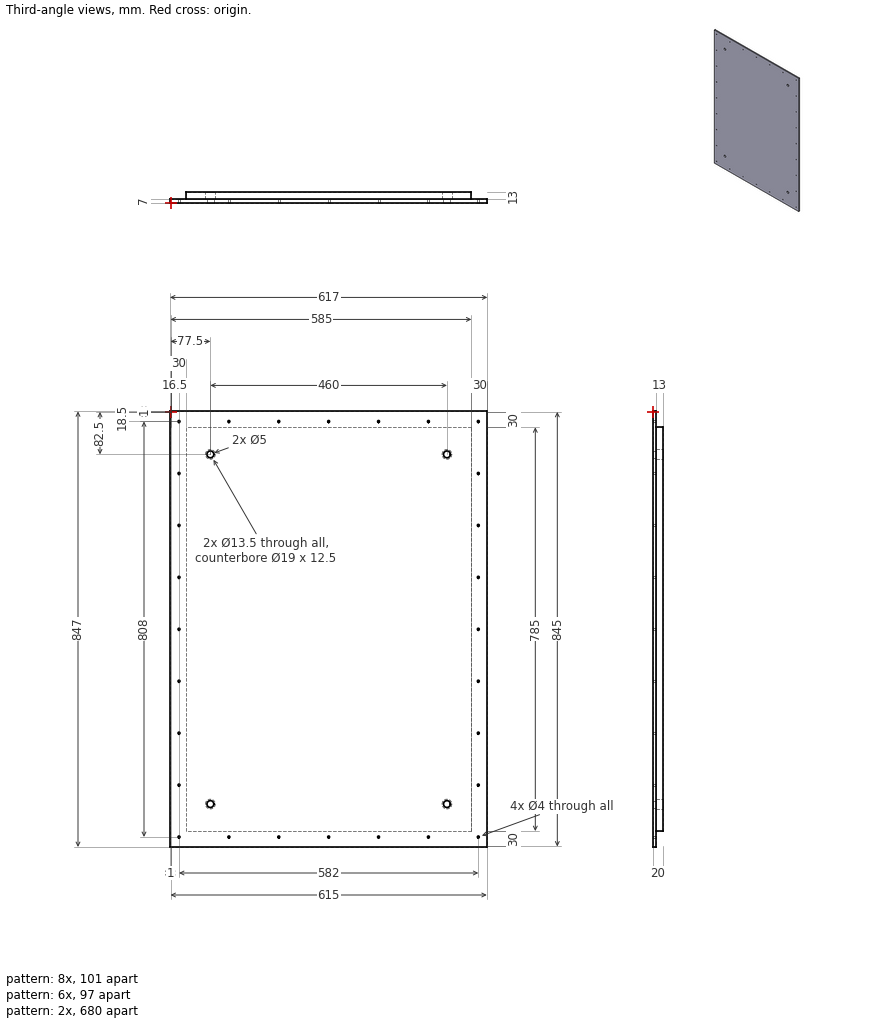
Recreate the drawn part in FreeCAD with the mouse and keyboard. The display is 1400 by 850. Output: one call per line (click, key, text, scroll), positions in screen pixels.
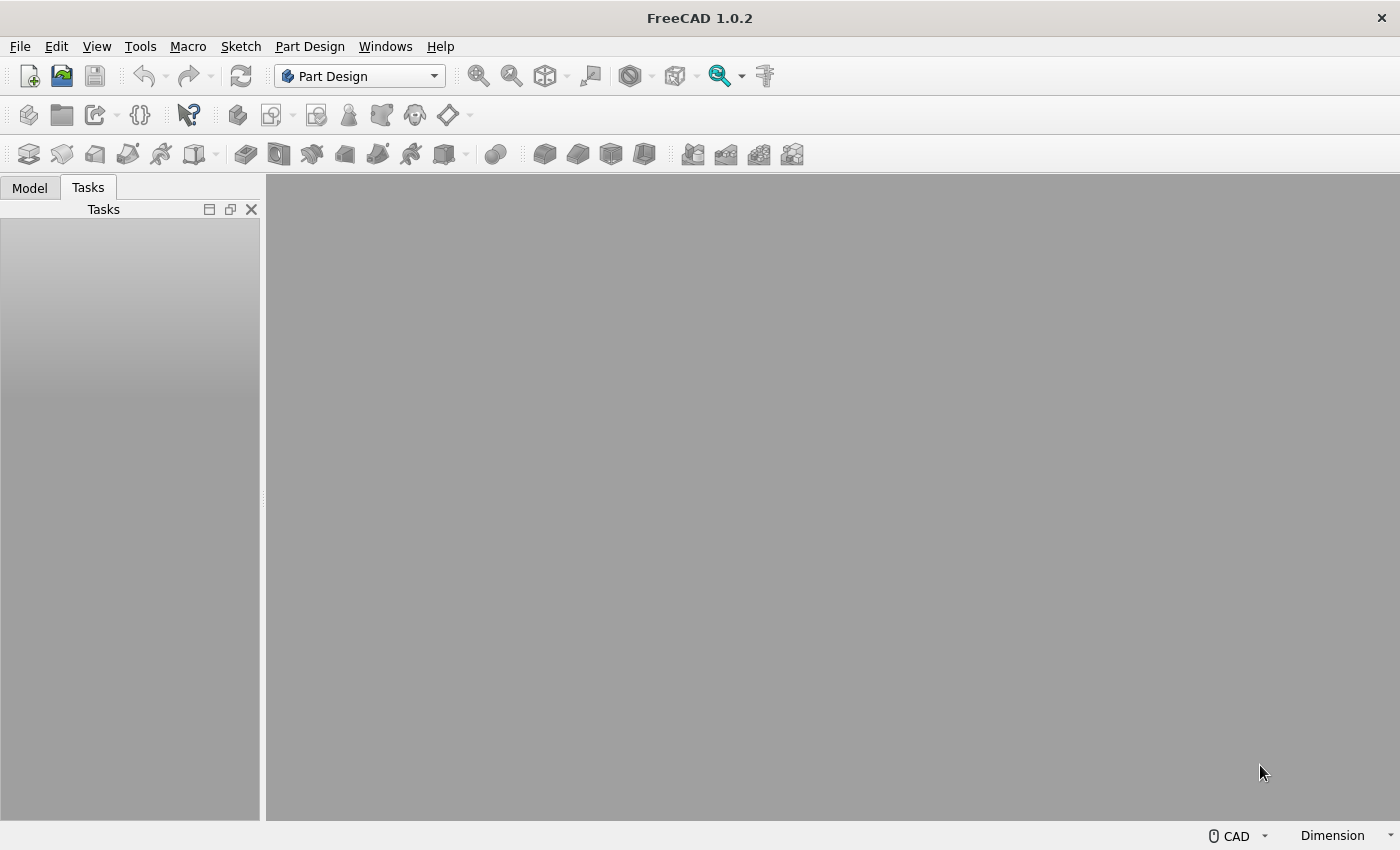
click(29, 76)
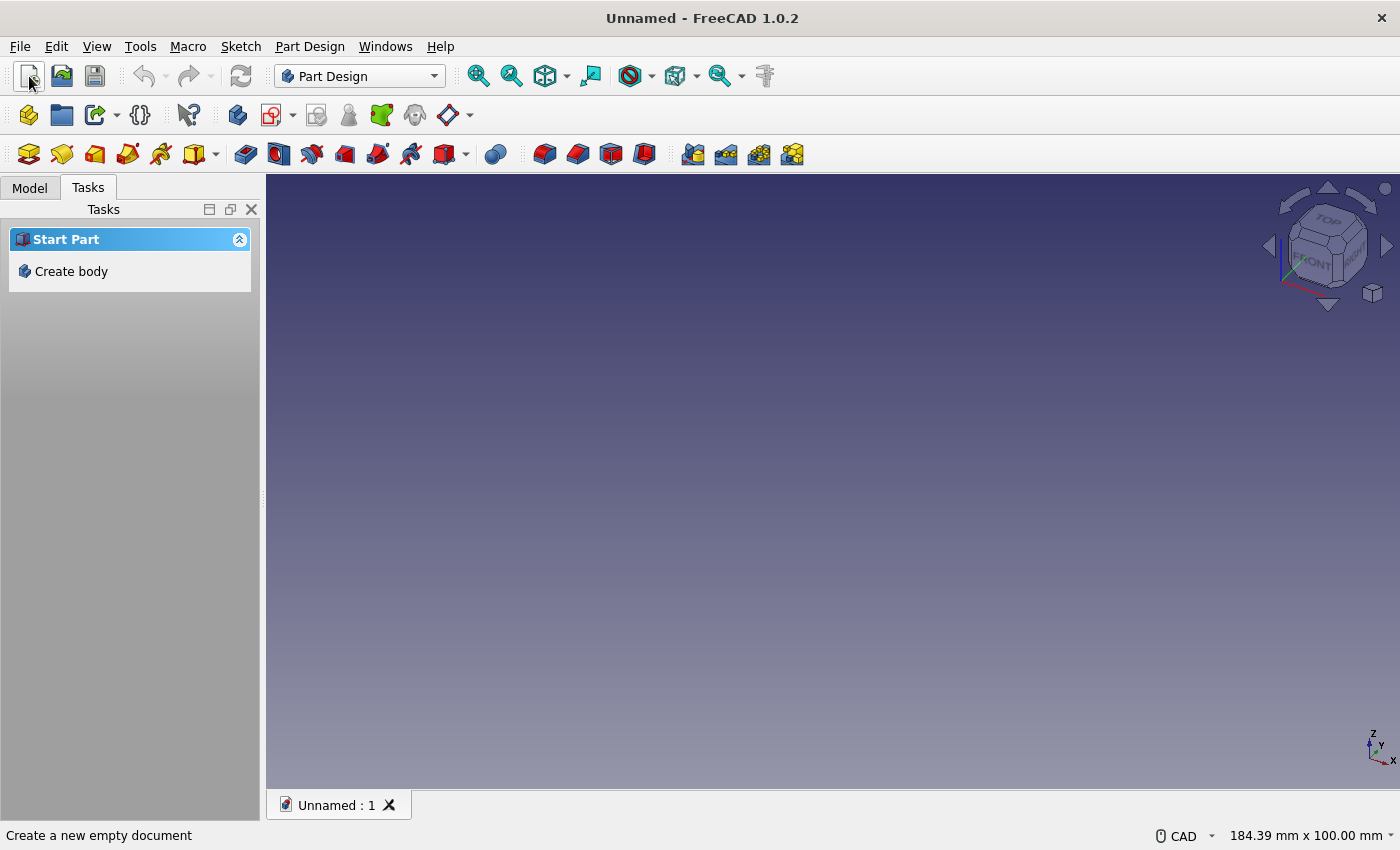
click(270, 116)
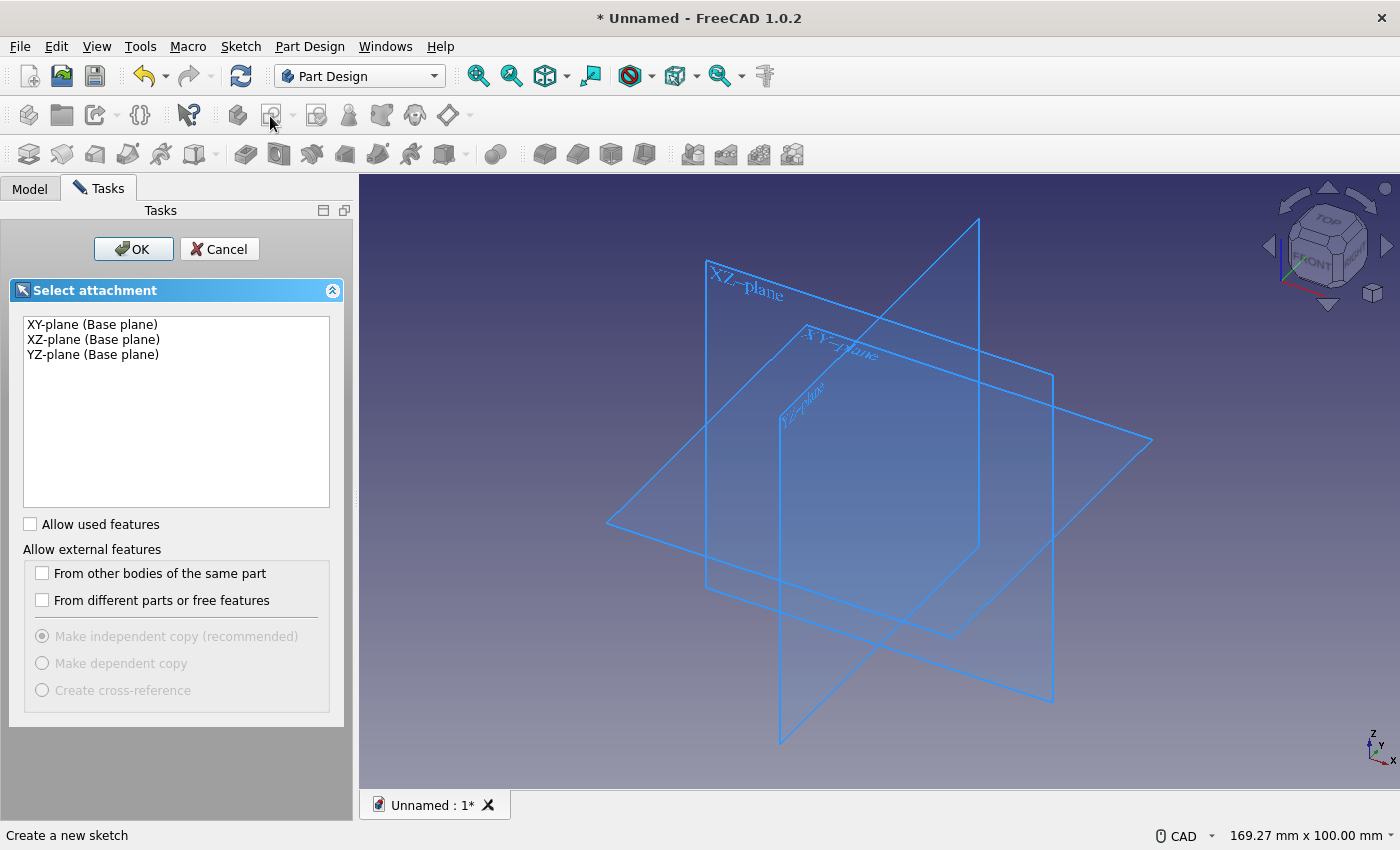
click(84, 340)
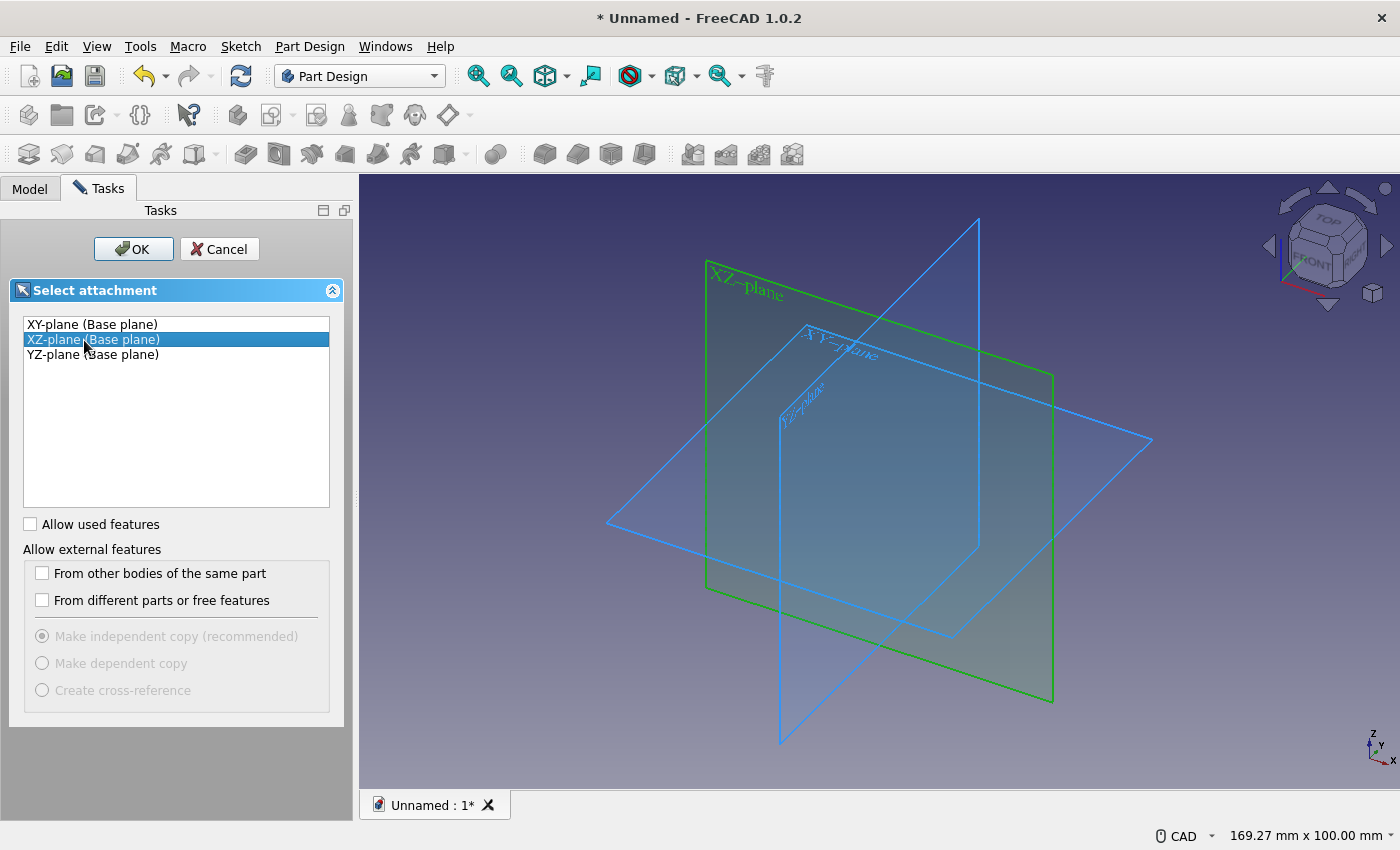
click(134, 249)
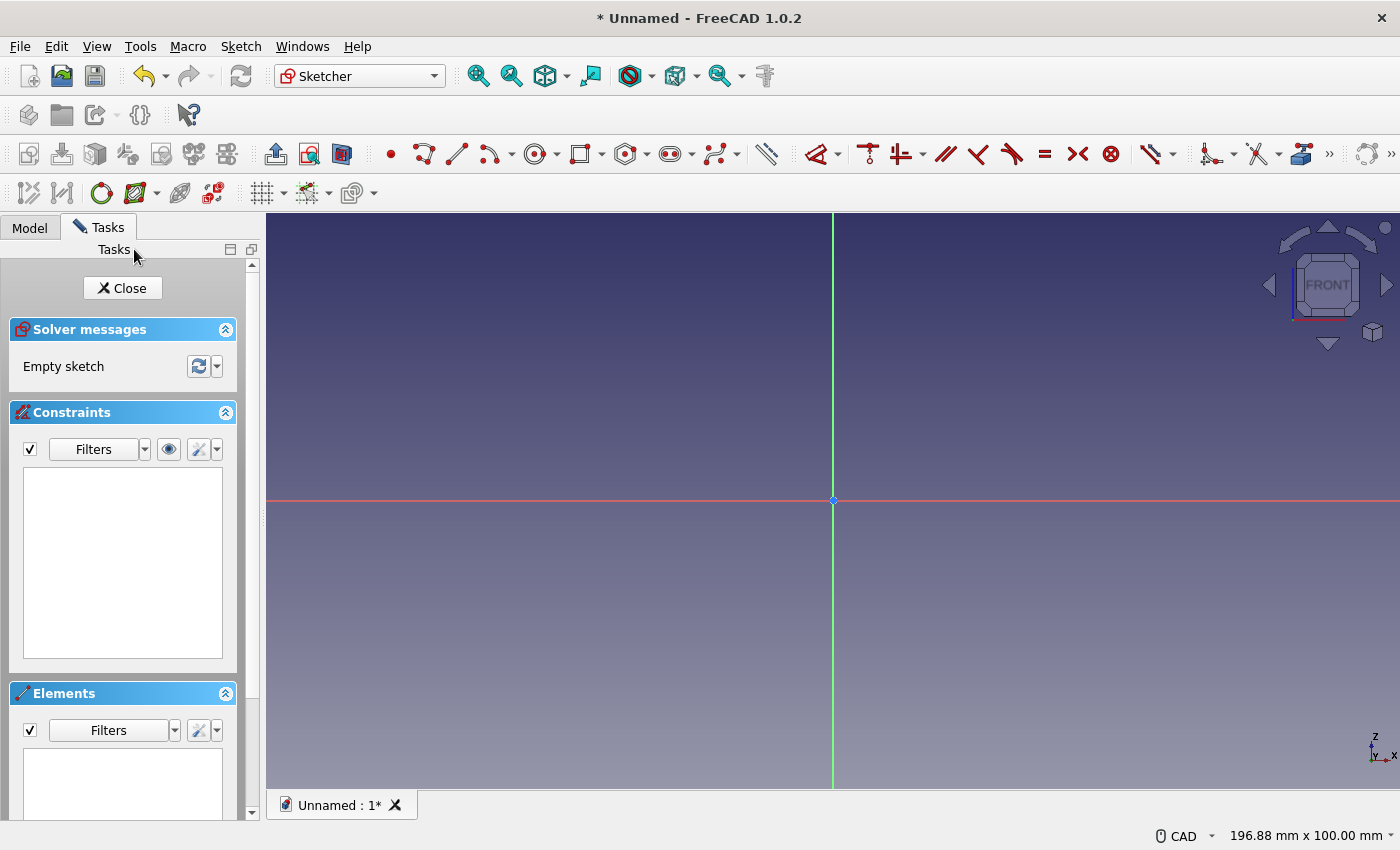
scroll(617, 306, down, 13)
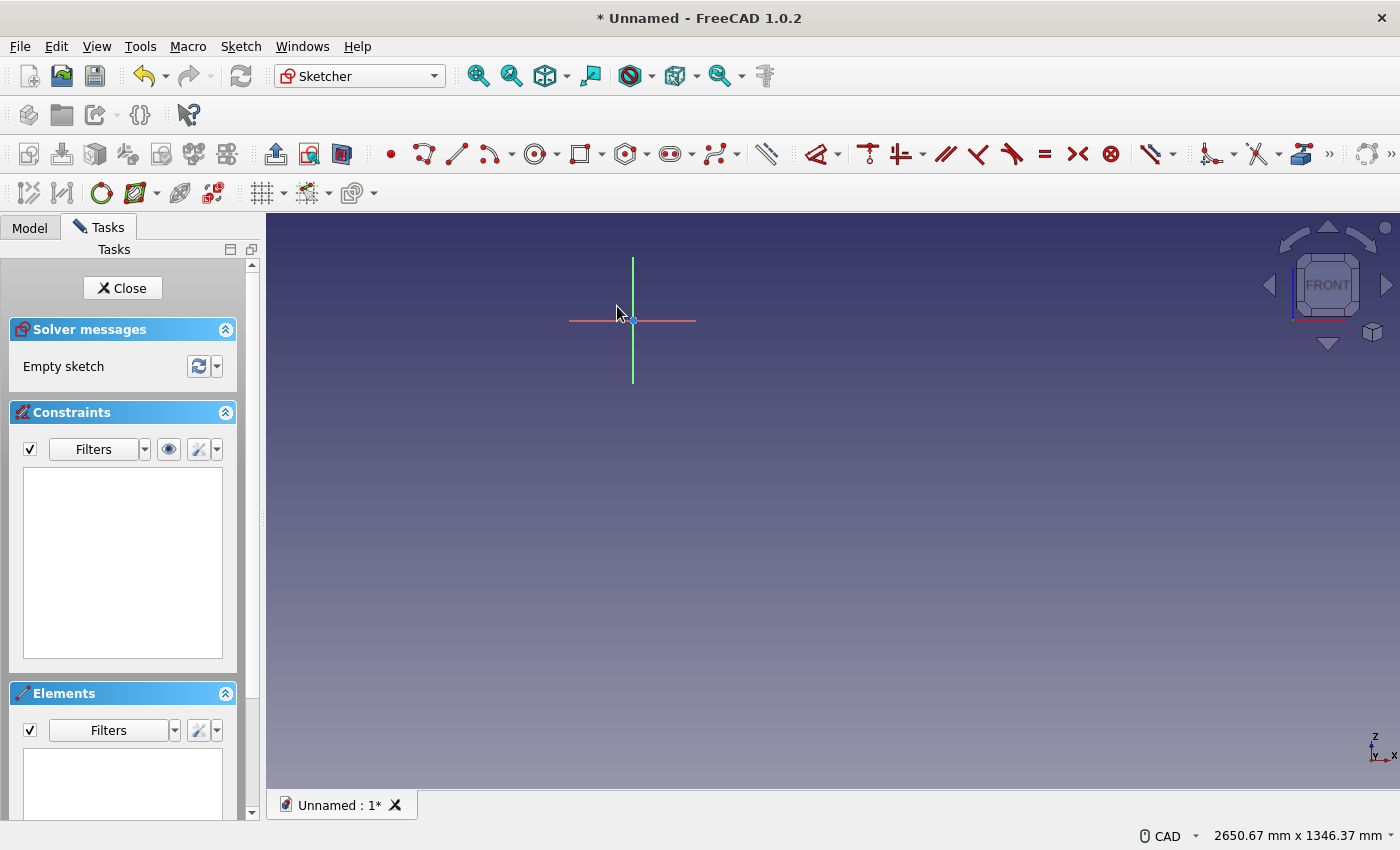
click(580, 154)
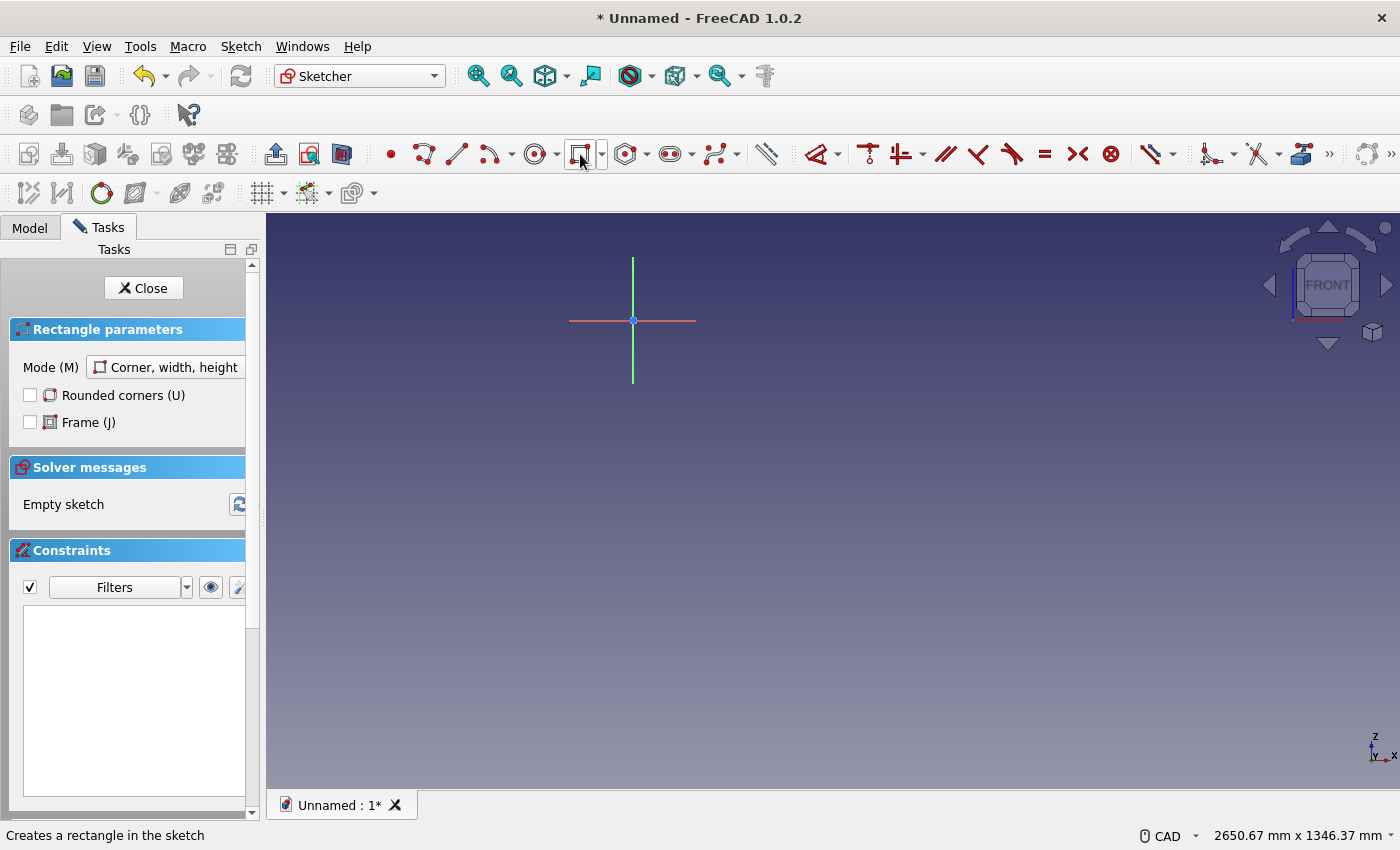
click(633, 321)
move(896, 682)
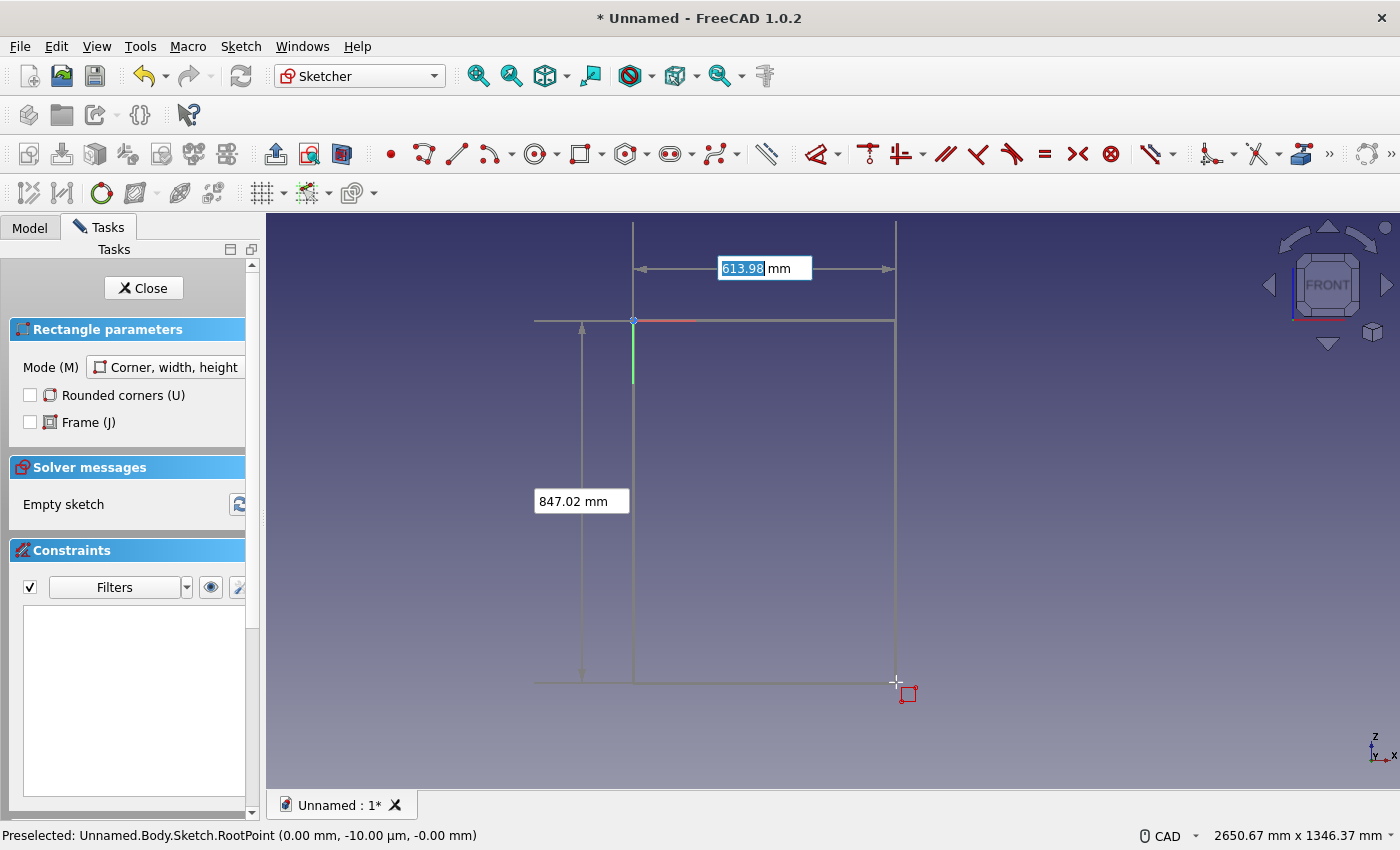
text(615)
key(Tab)
text(845)
key(Return)
key(Escape)